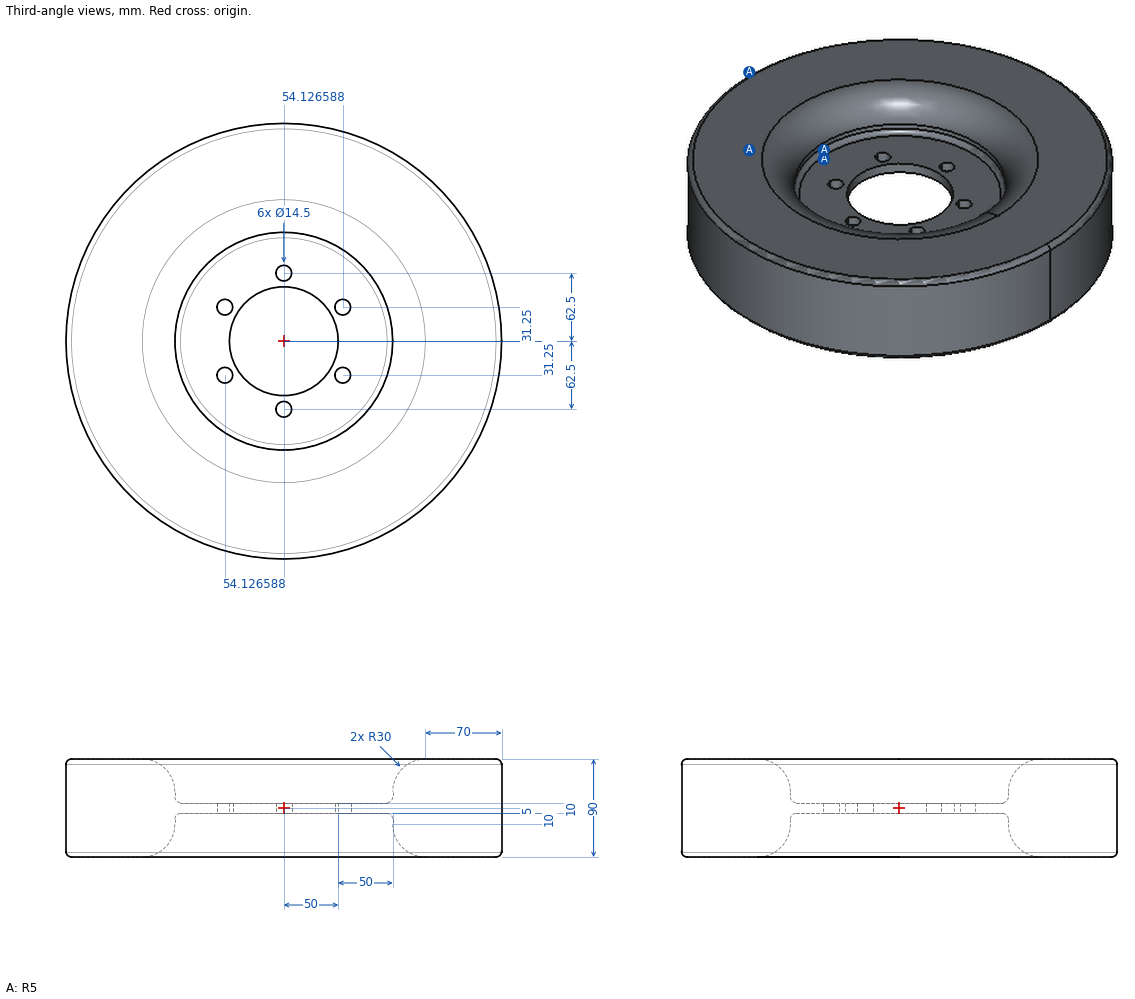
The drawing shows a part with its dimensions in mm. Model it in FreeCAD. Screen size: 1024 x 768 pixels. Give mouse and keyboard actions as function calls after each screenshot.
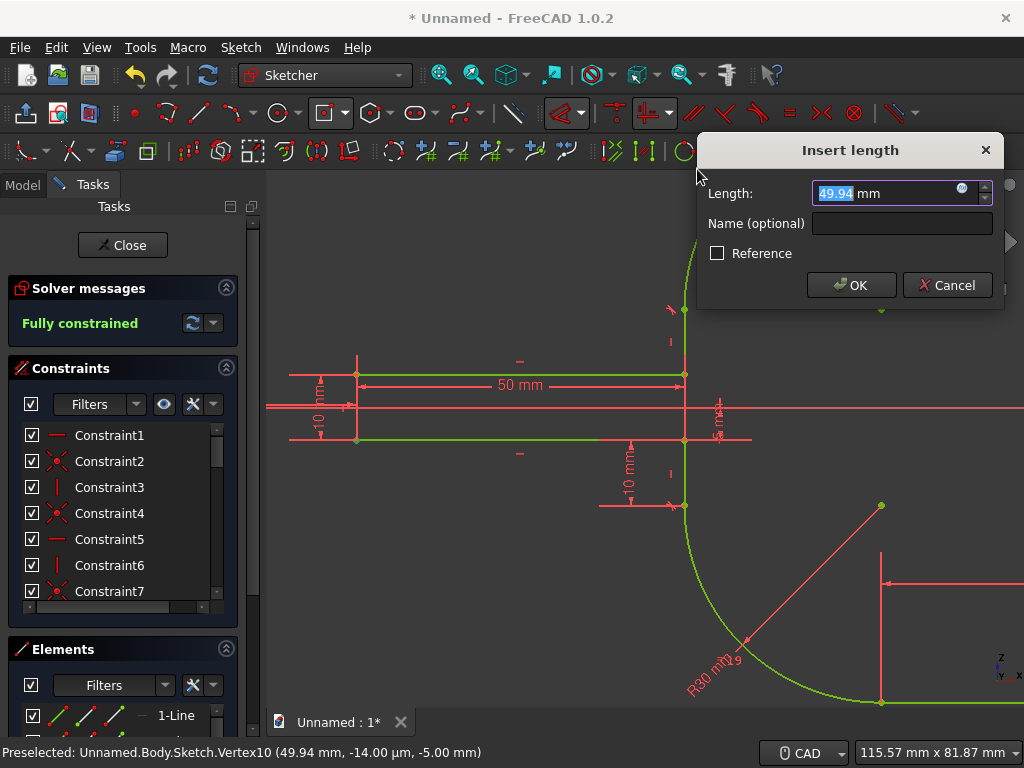
text(50)
key(Return)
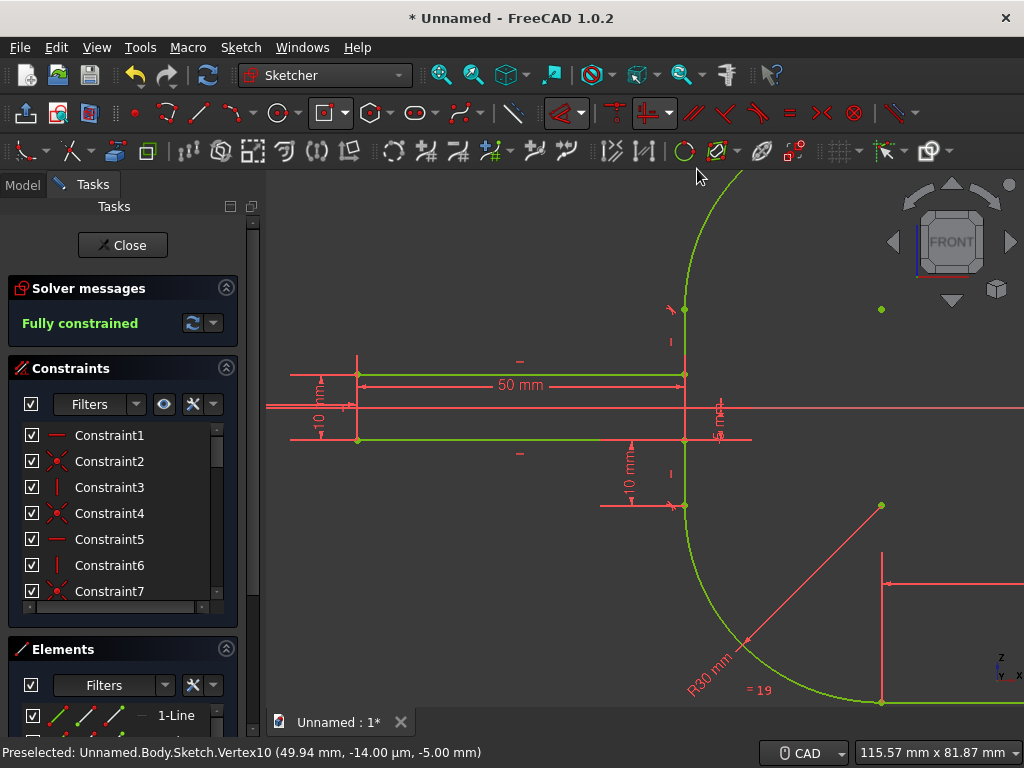
click(123, 245)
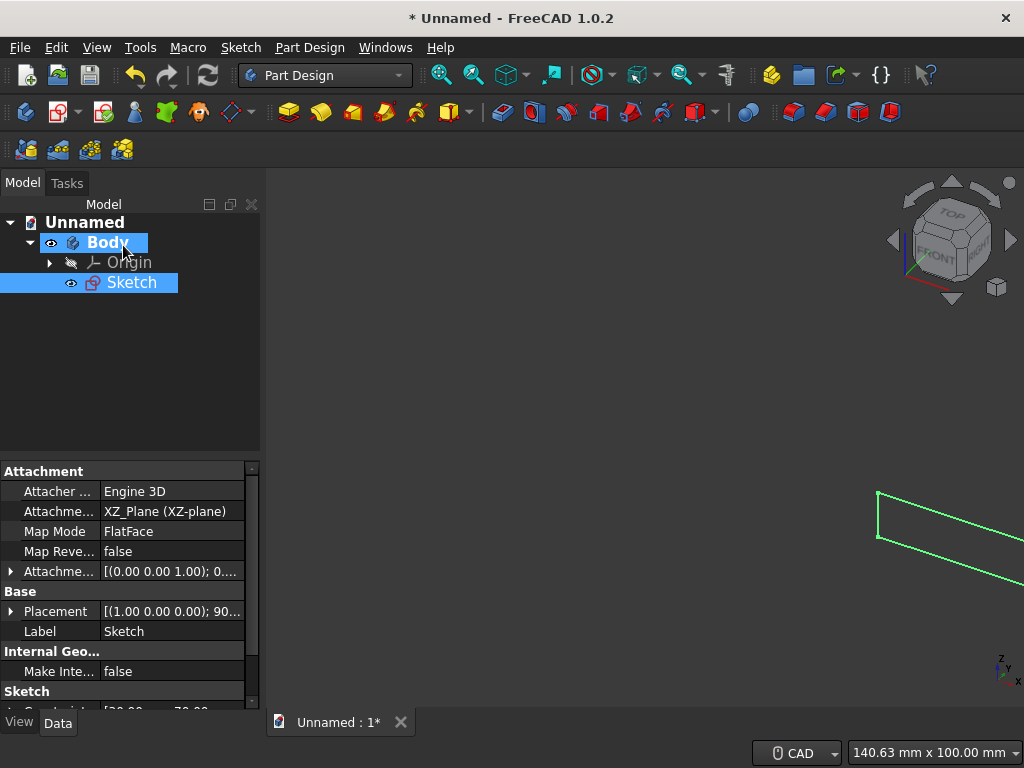
click(322, 112)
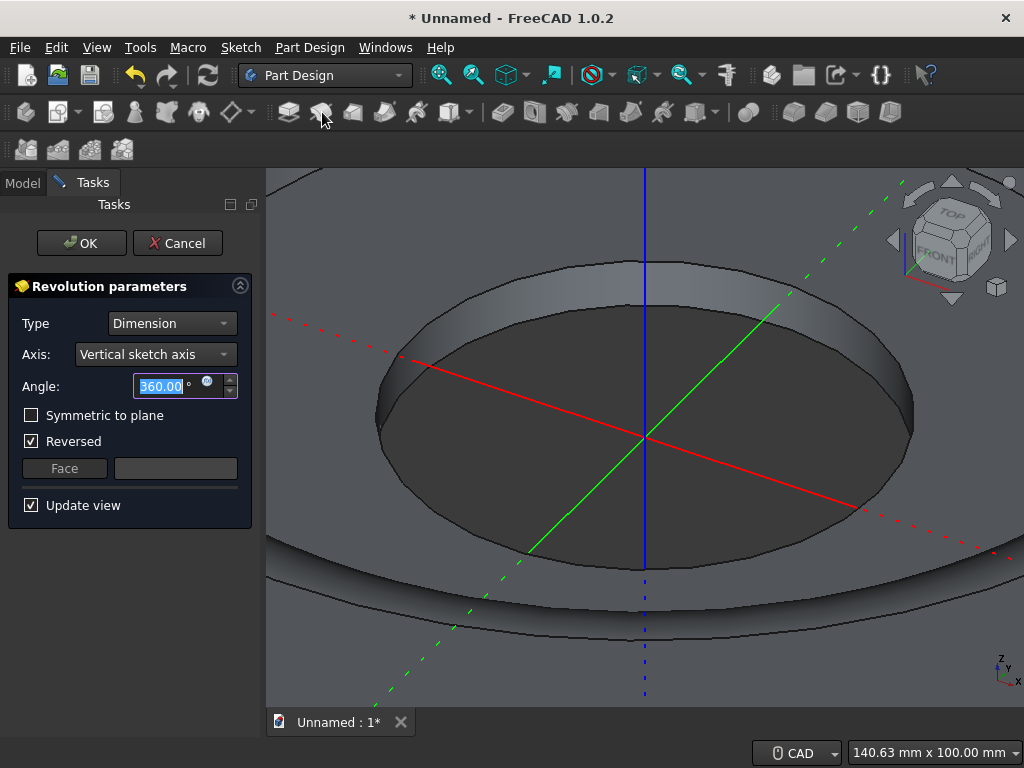
click(82, 243)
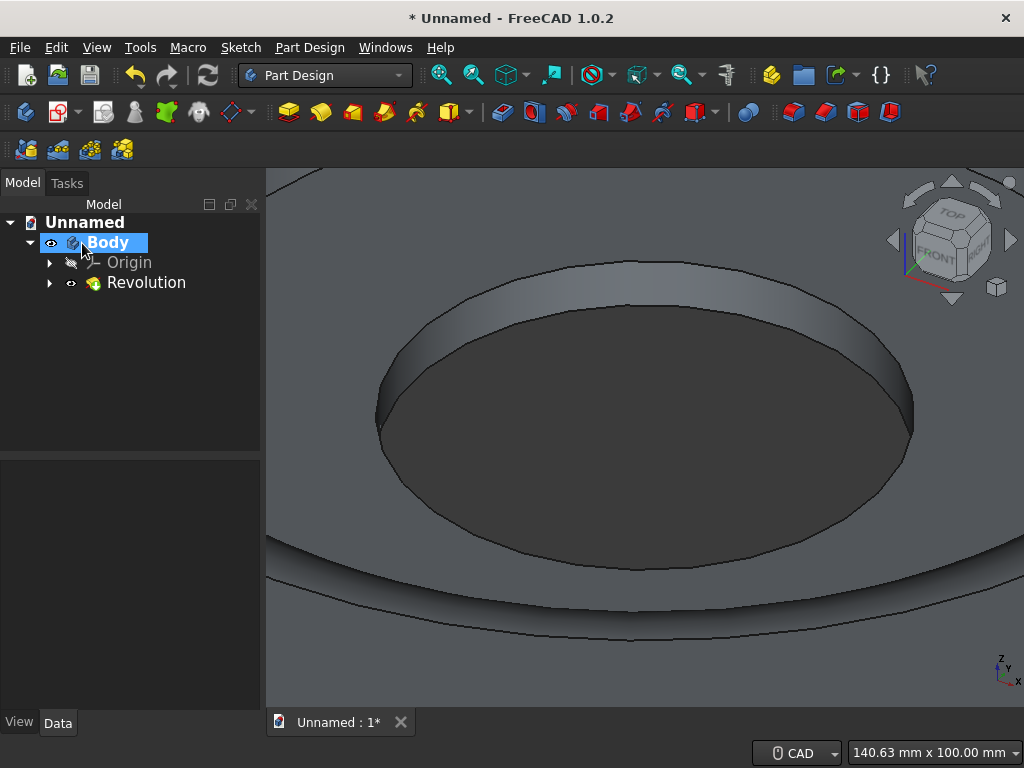
click(442, 76)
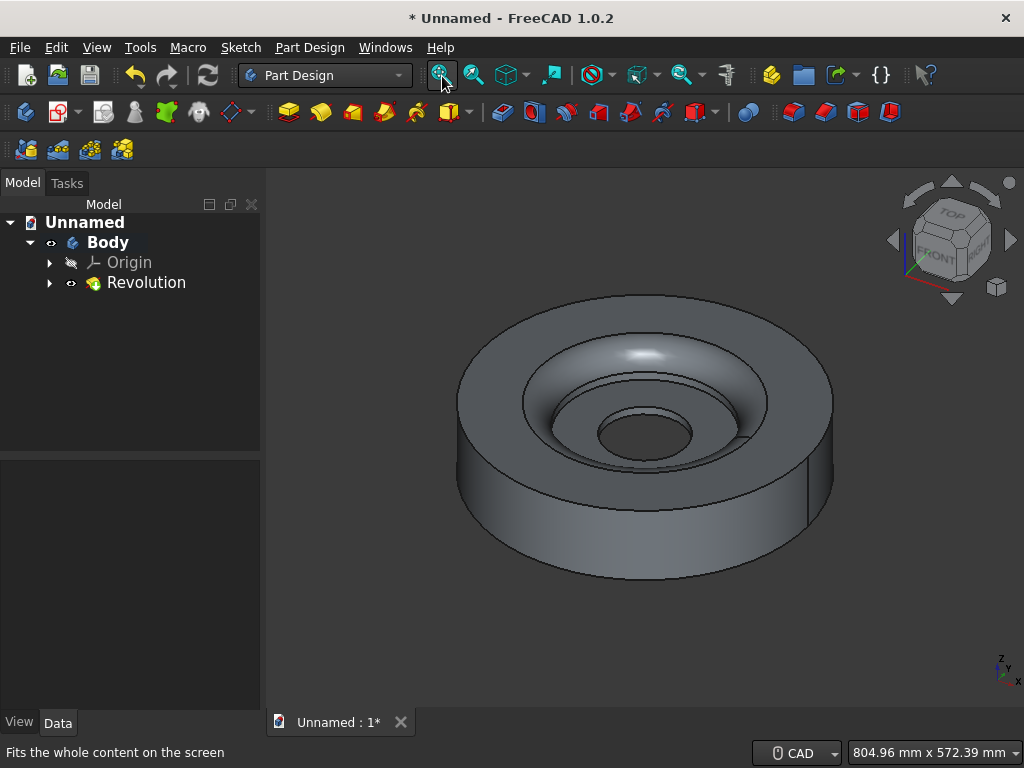
click(458, 413)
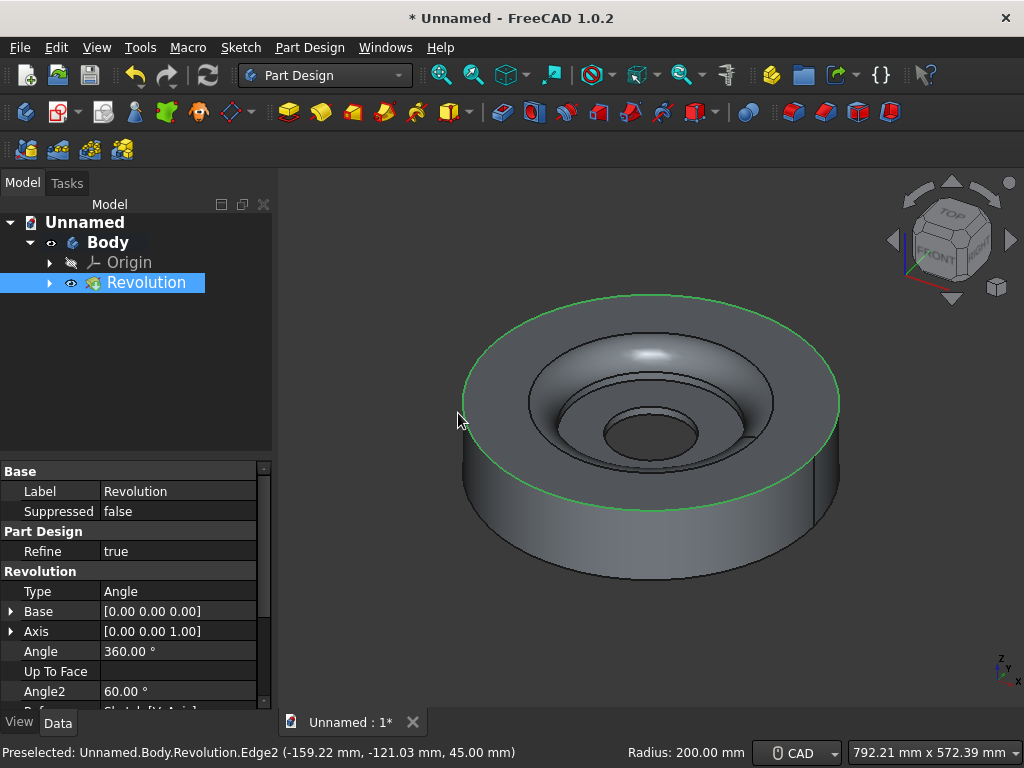
key(0)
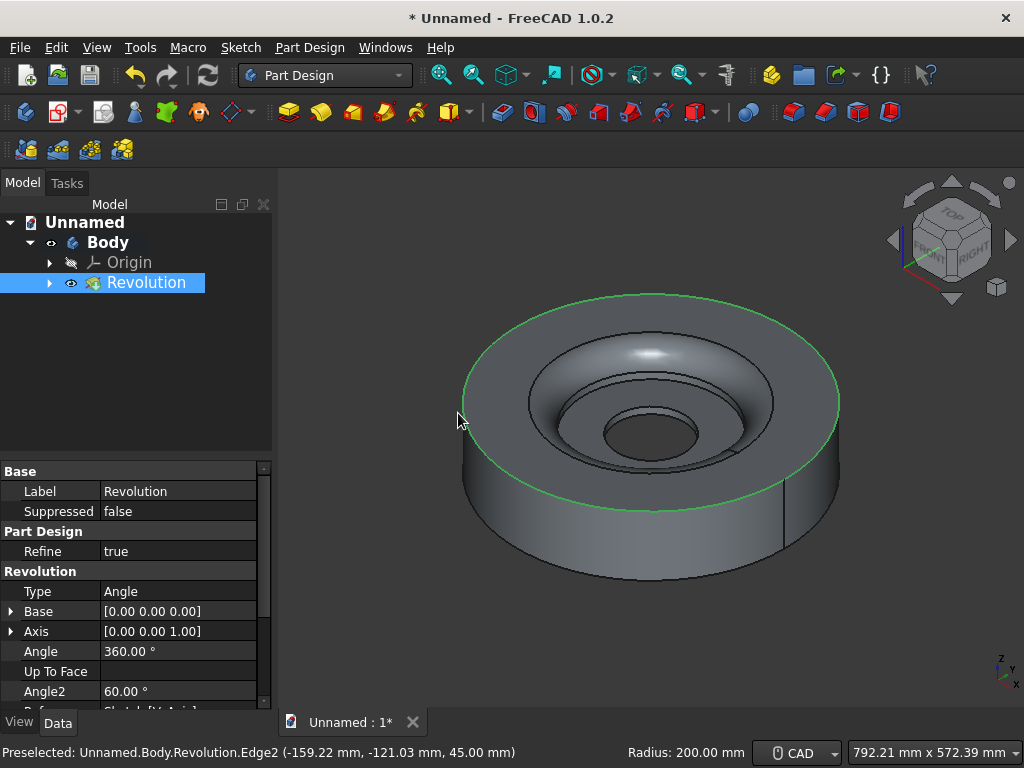
key(2)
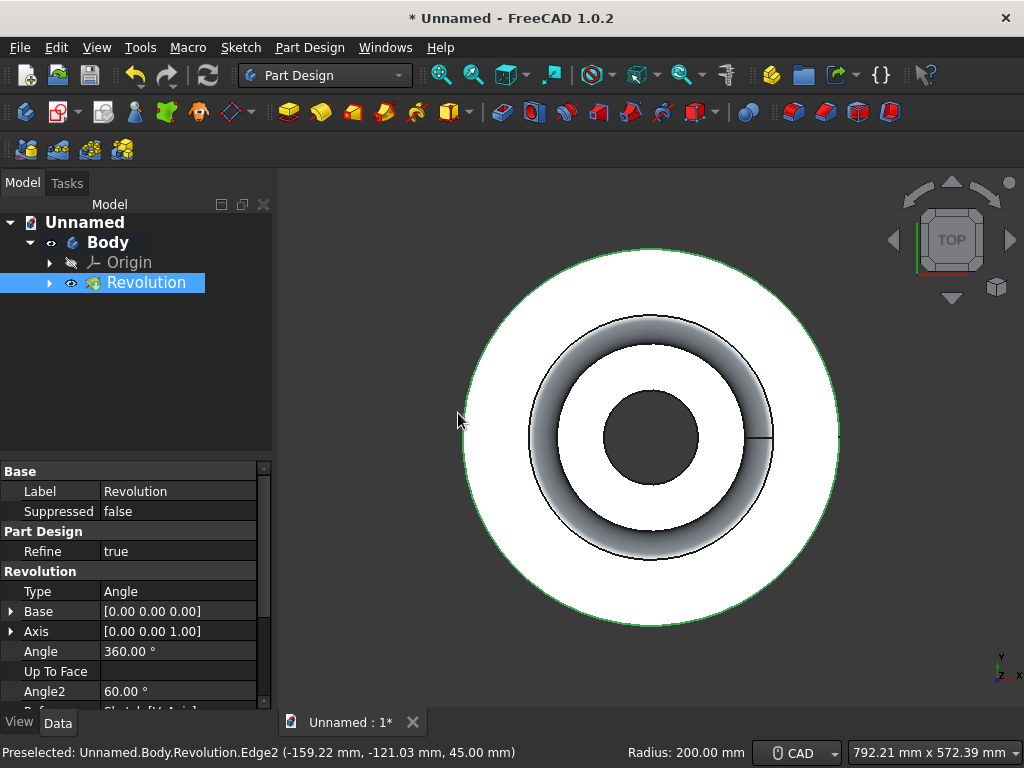
key(1)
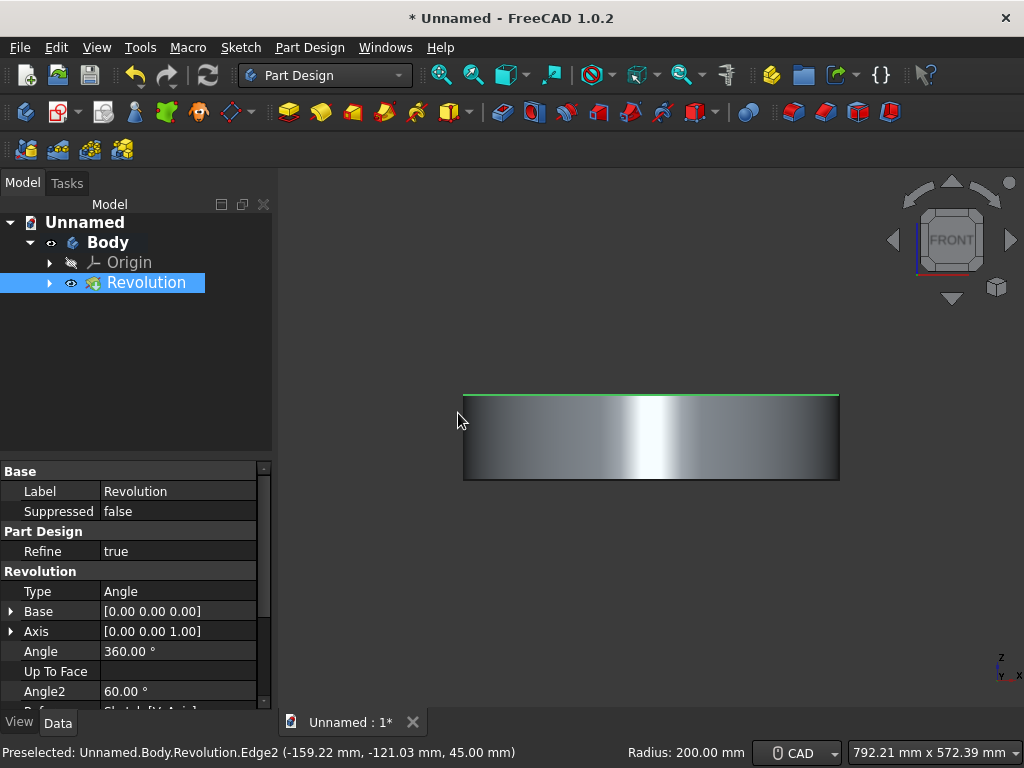
click(499, 479, ctrl)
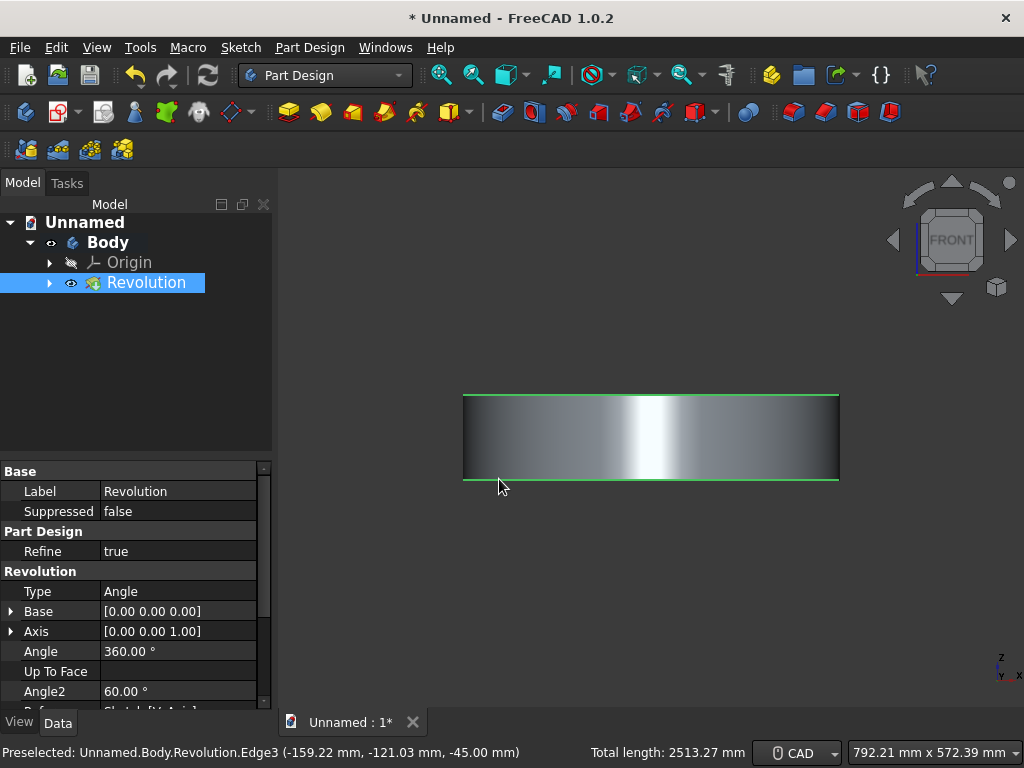
key(3)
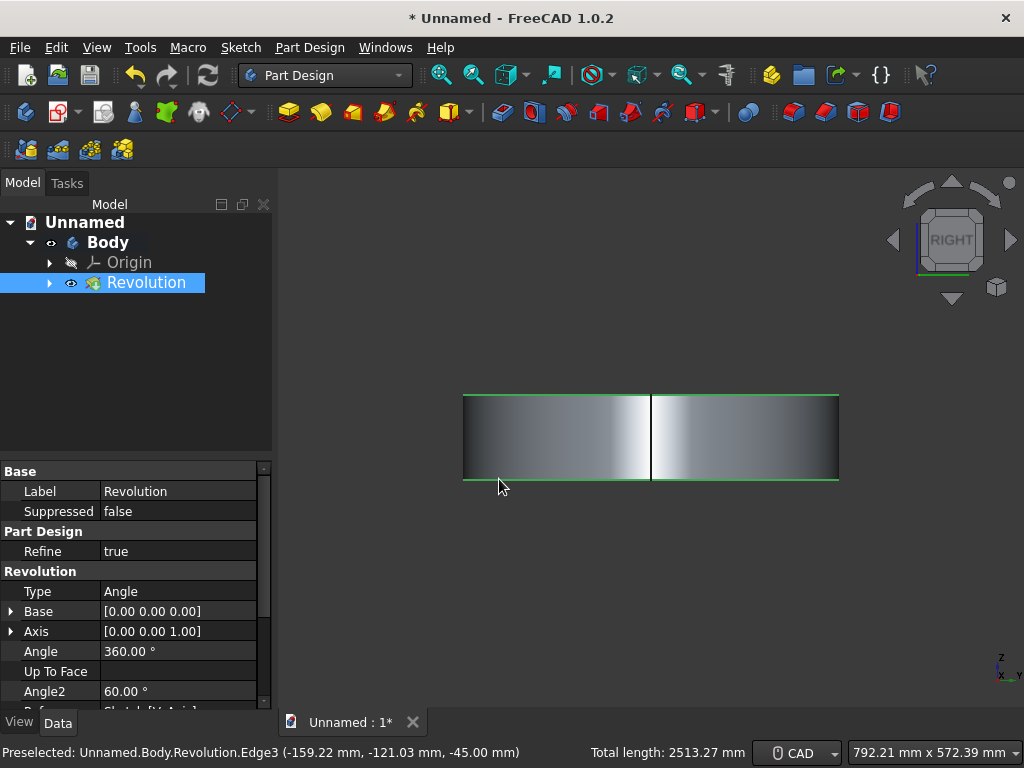
key(5)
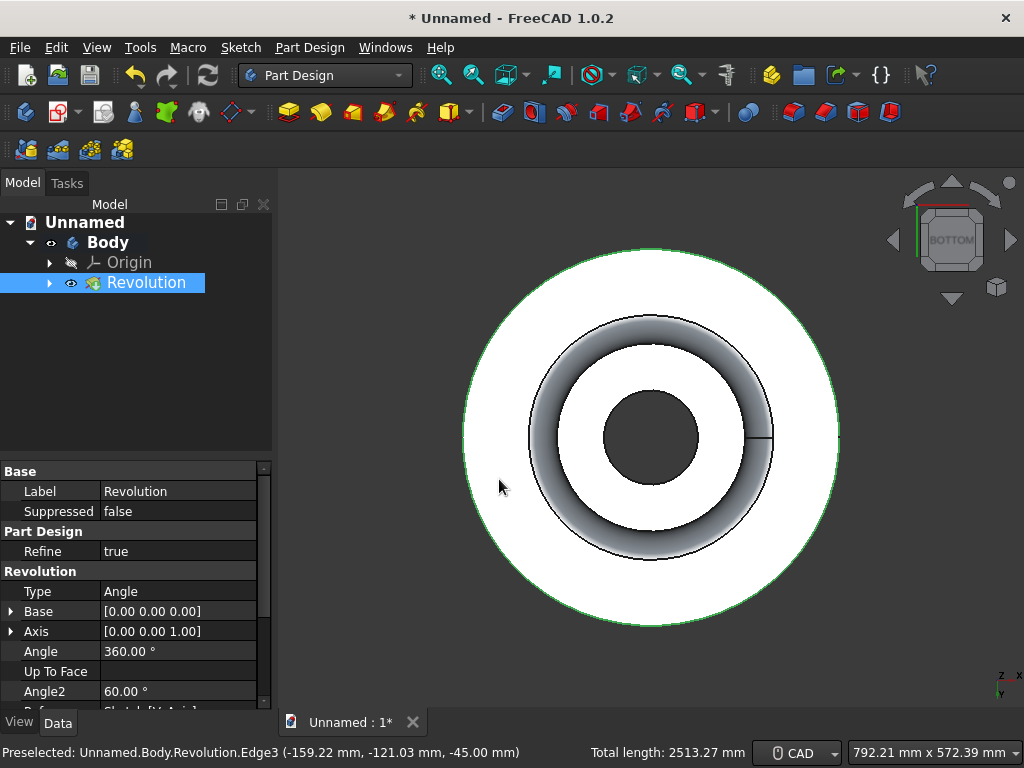
key(4)